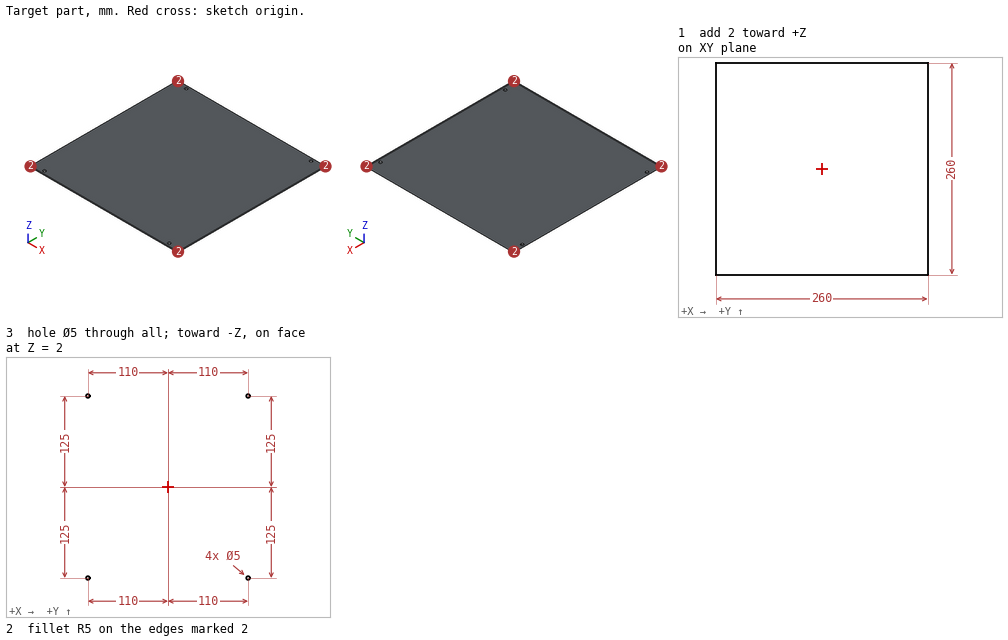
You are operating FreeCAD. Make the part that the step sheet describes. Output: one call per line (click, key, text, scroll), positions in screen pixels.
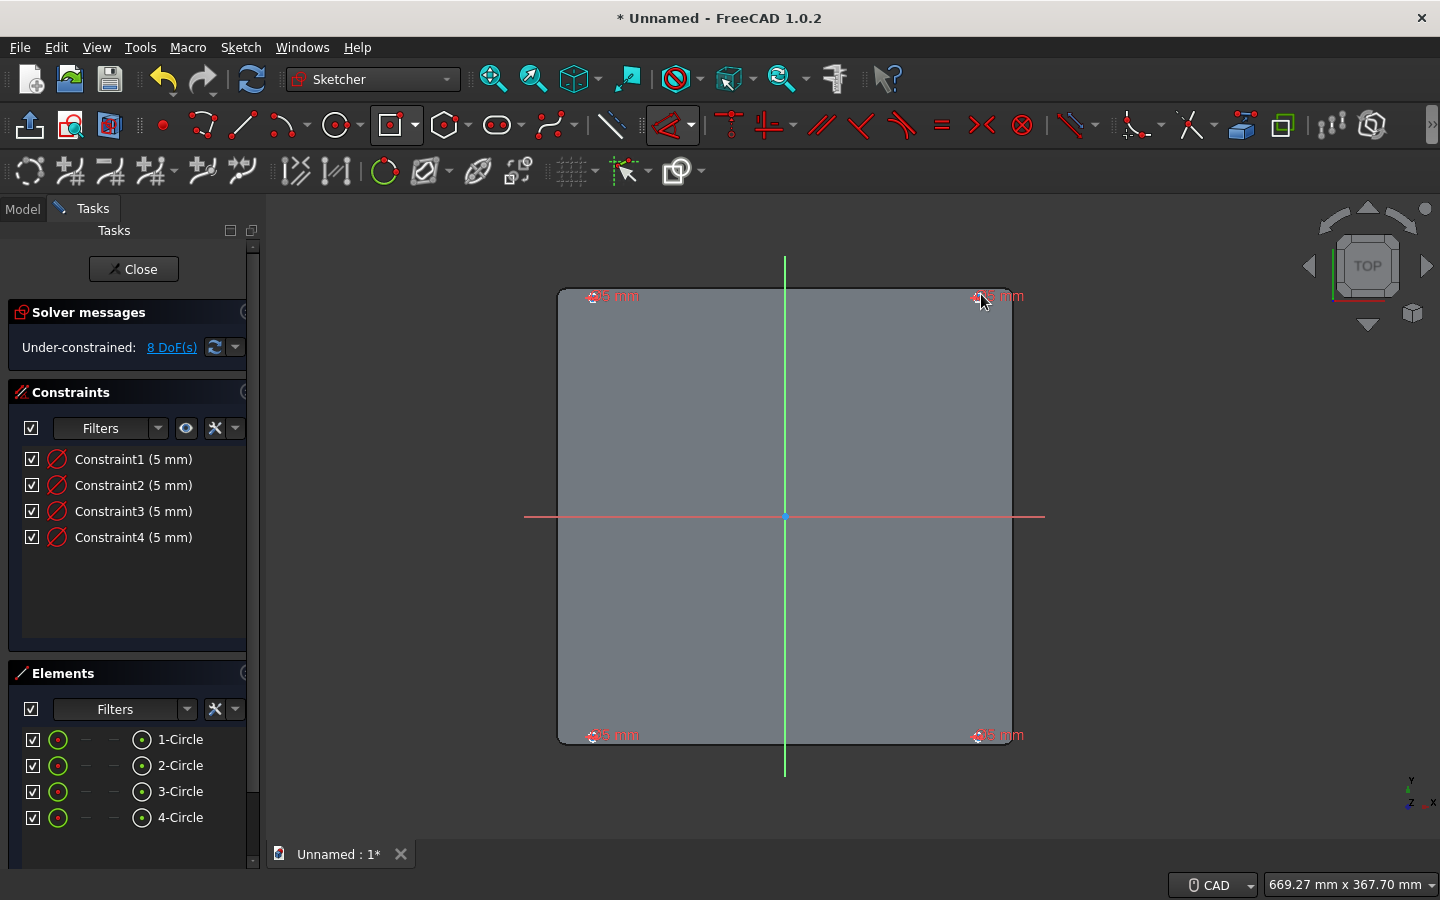
click(593, 298)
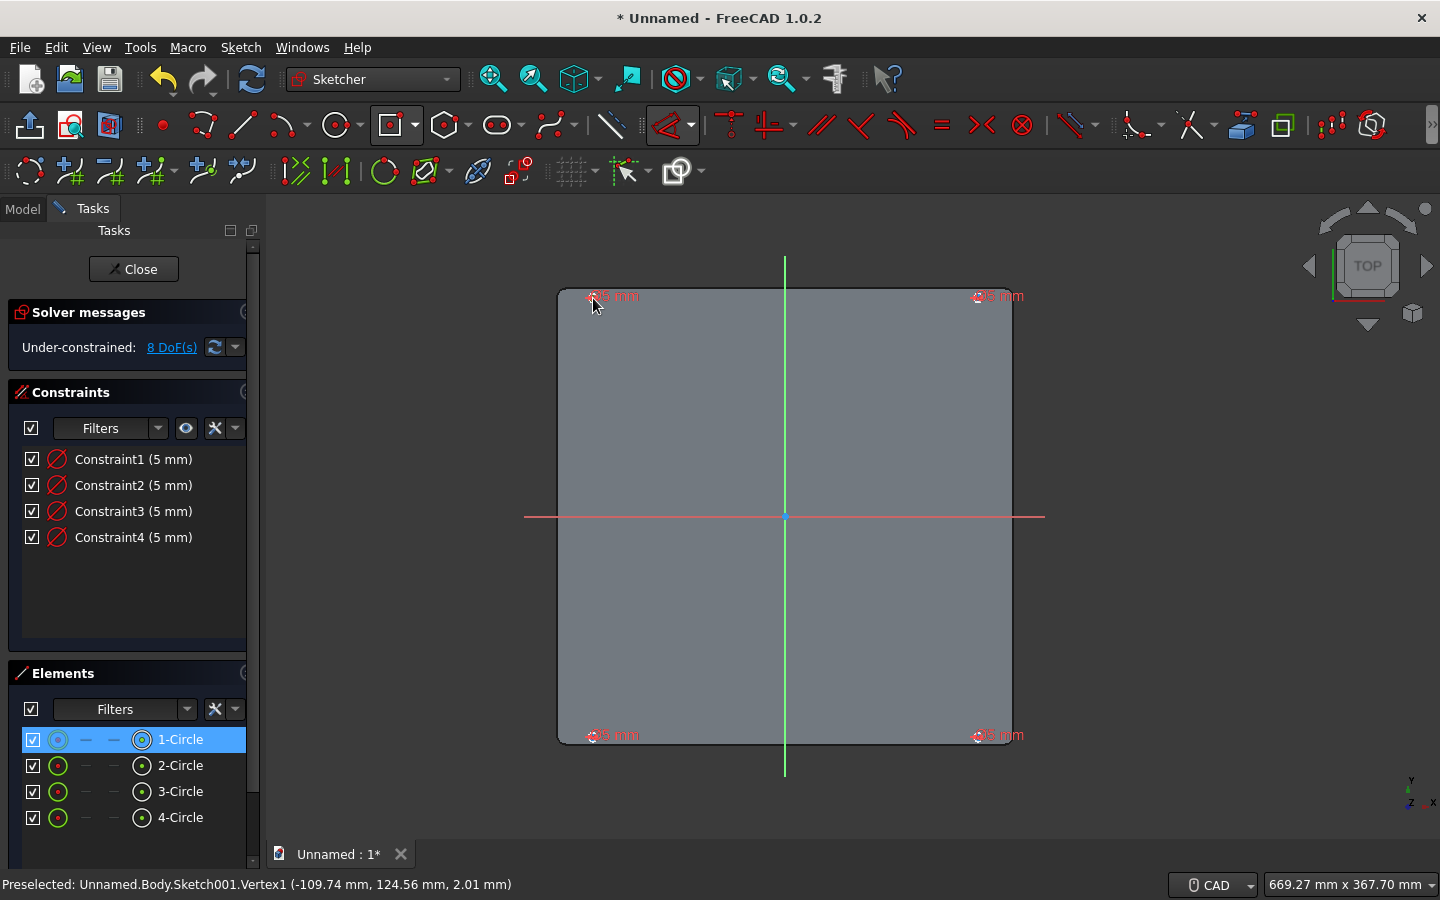
key(l)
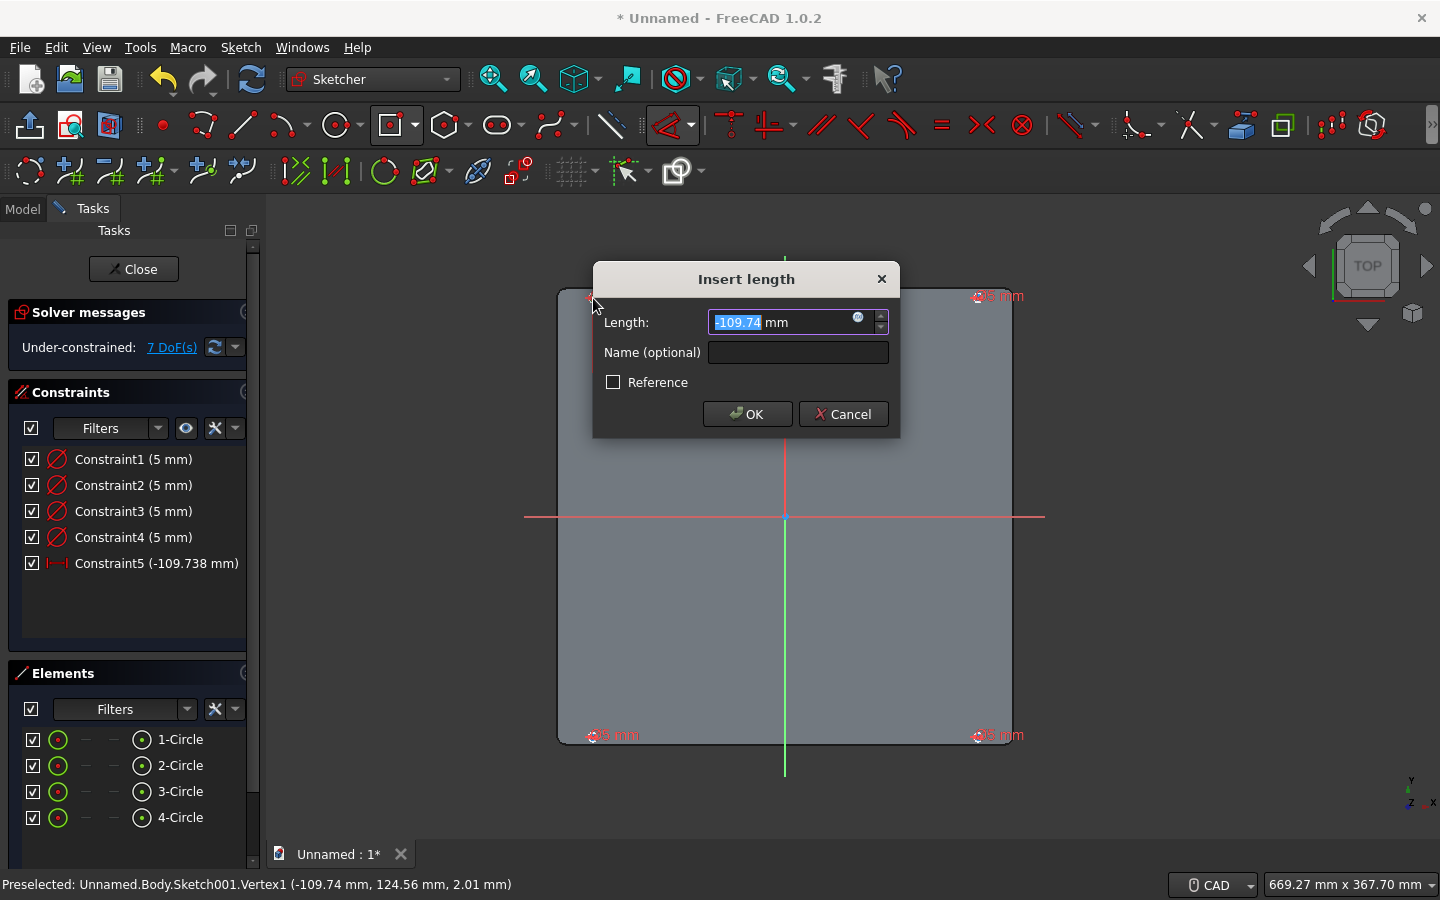
text(-110)
key(Return)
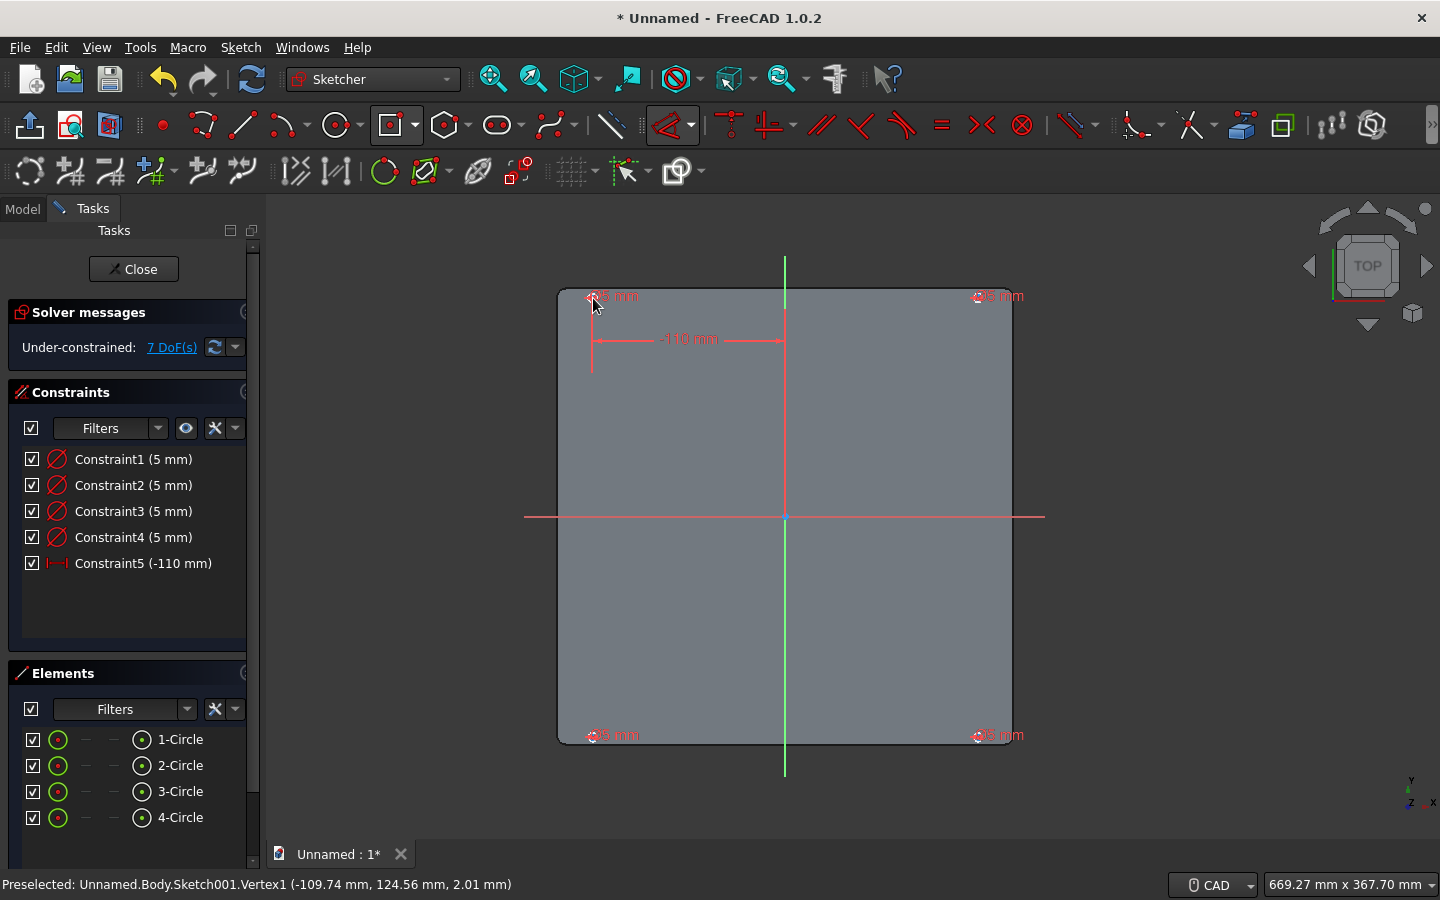
click(592, 298)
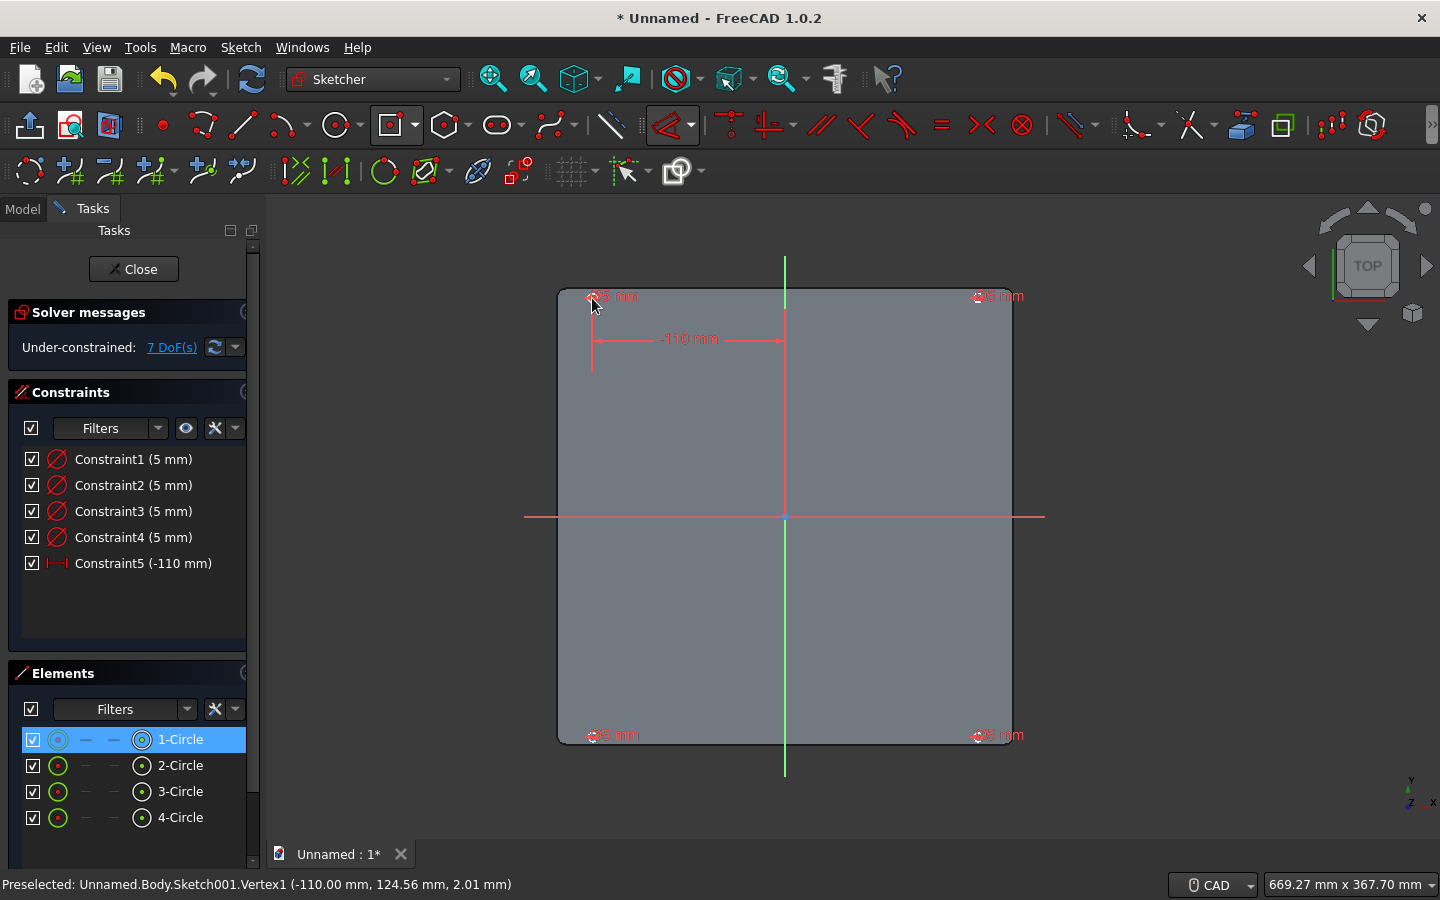
click(694, 126)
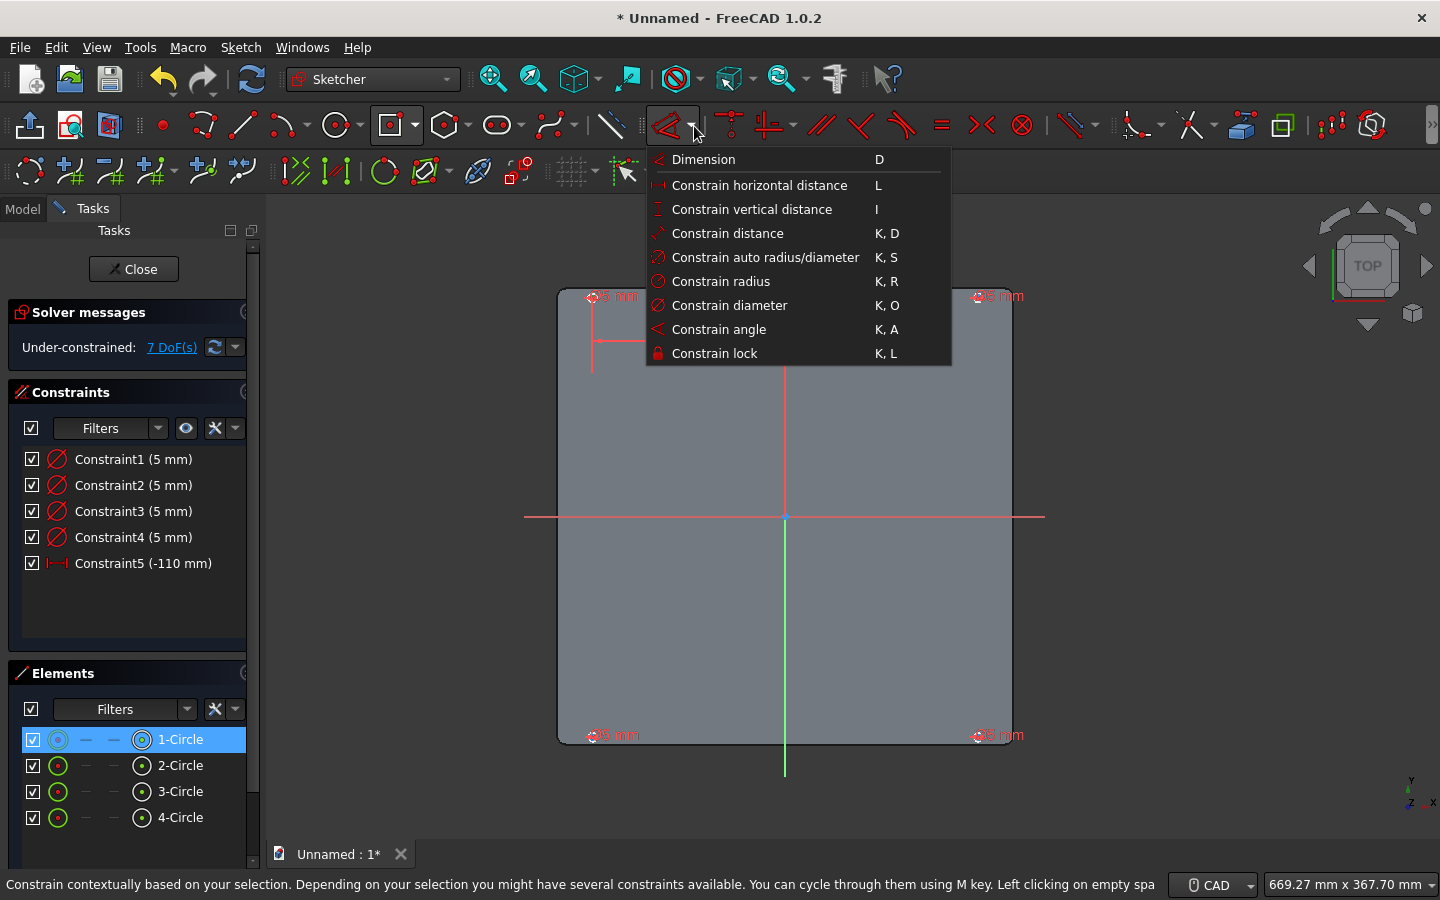
click(799, 209)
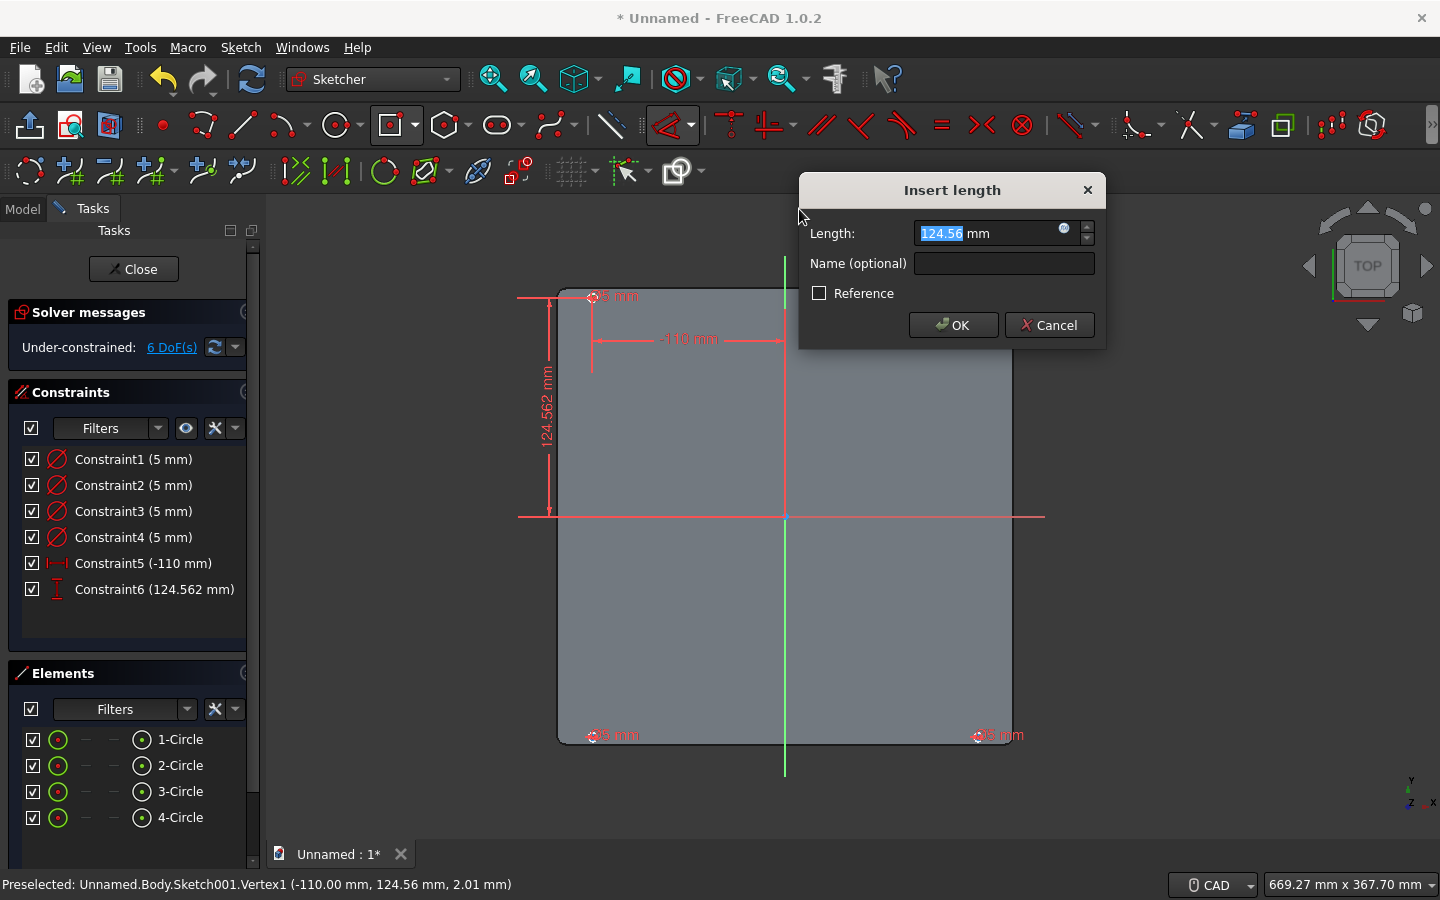
text(125)
key(Return)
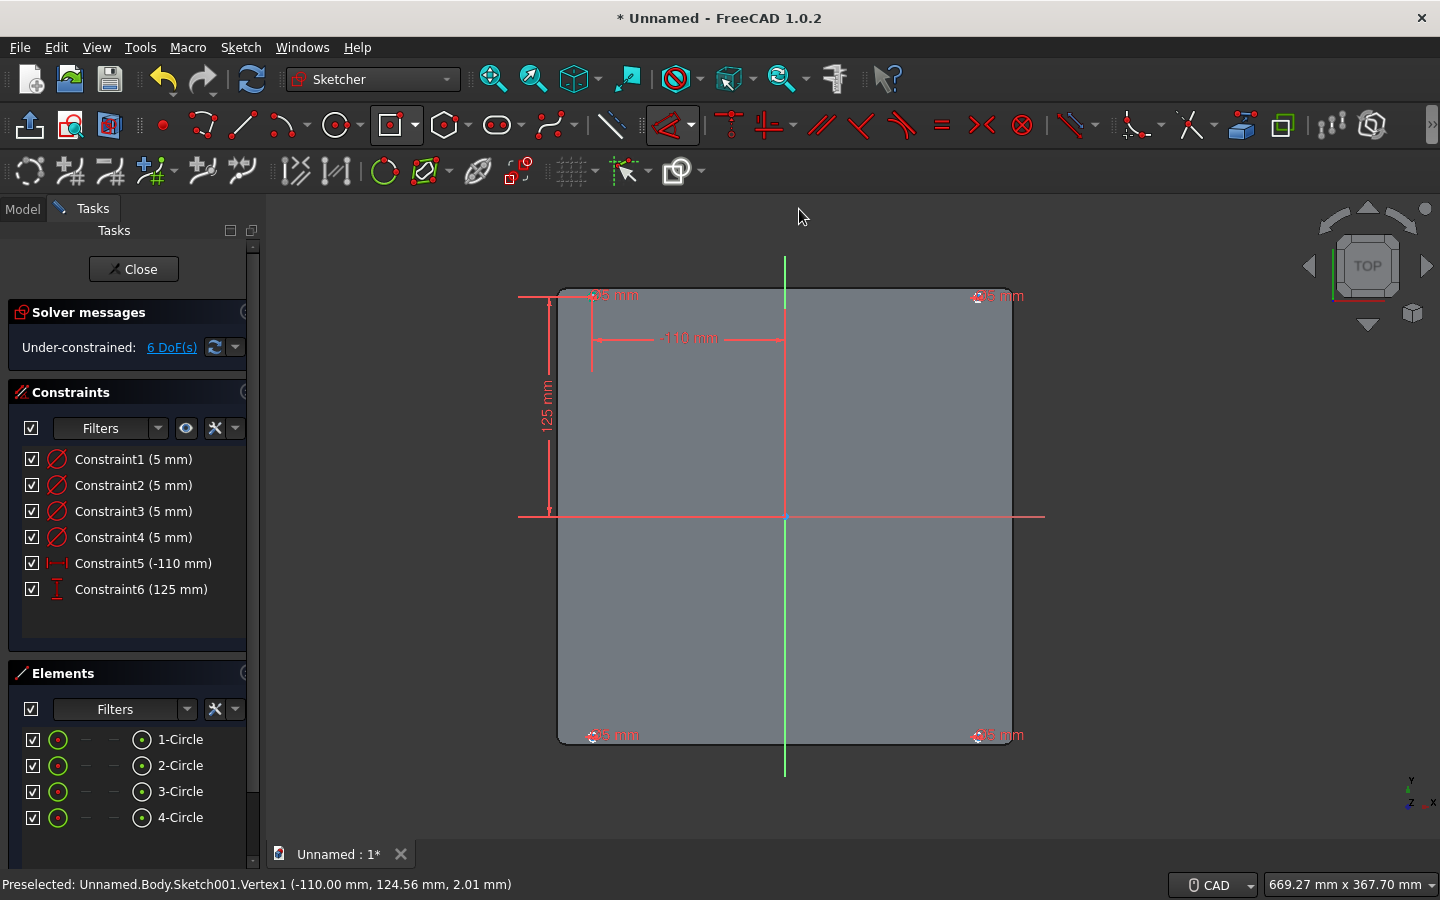
click(593, 737)